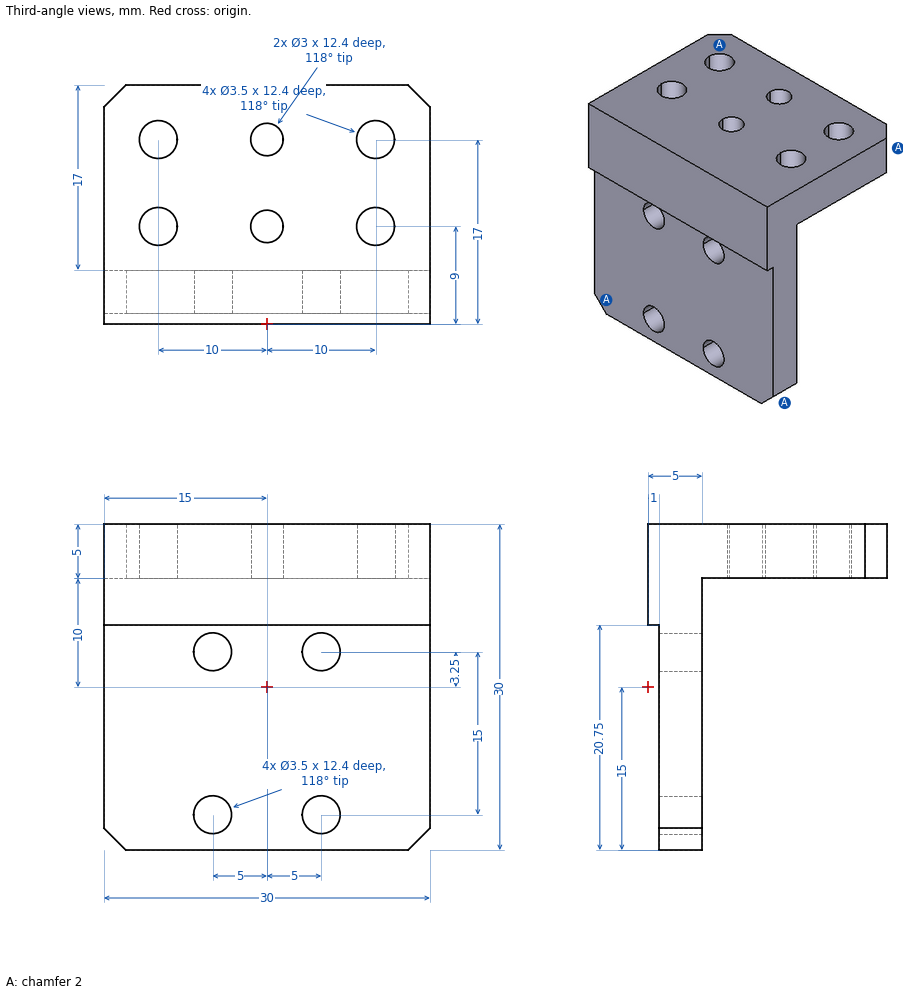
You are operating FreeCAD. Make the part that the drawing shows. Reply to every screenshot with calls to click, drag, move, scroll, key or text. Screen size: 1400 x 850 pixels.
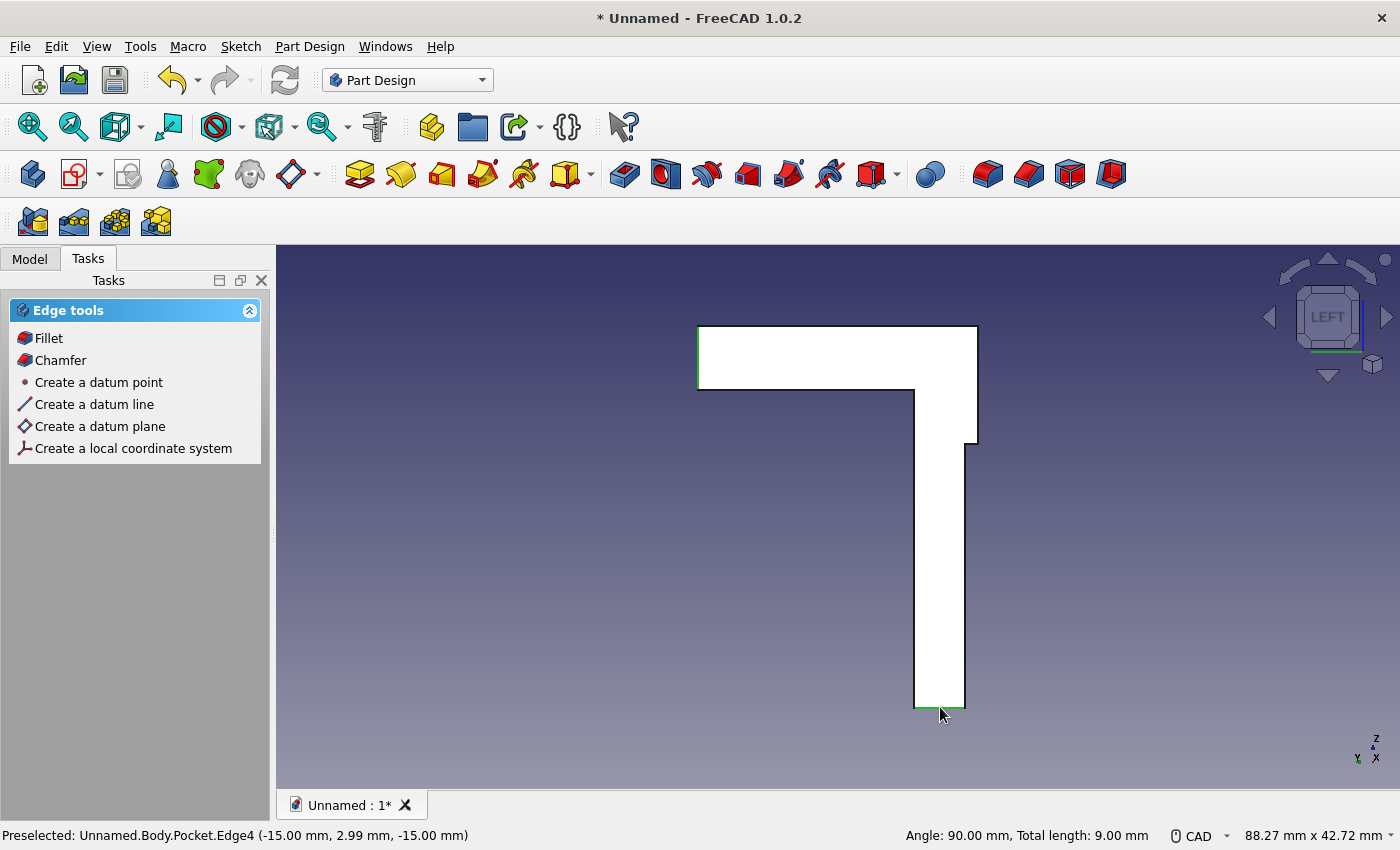
key(0)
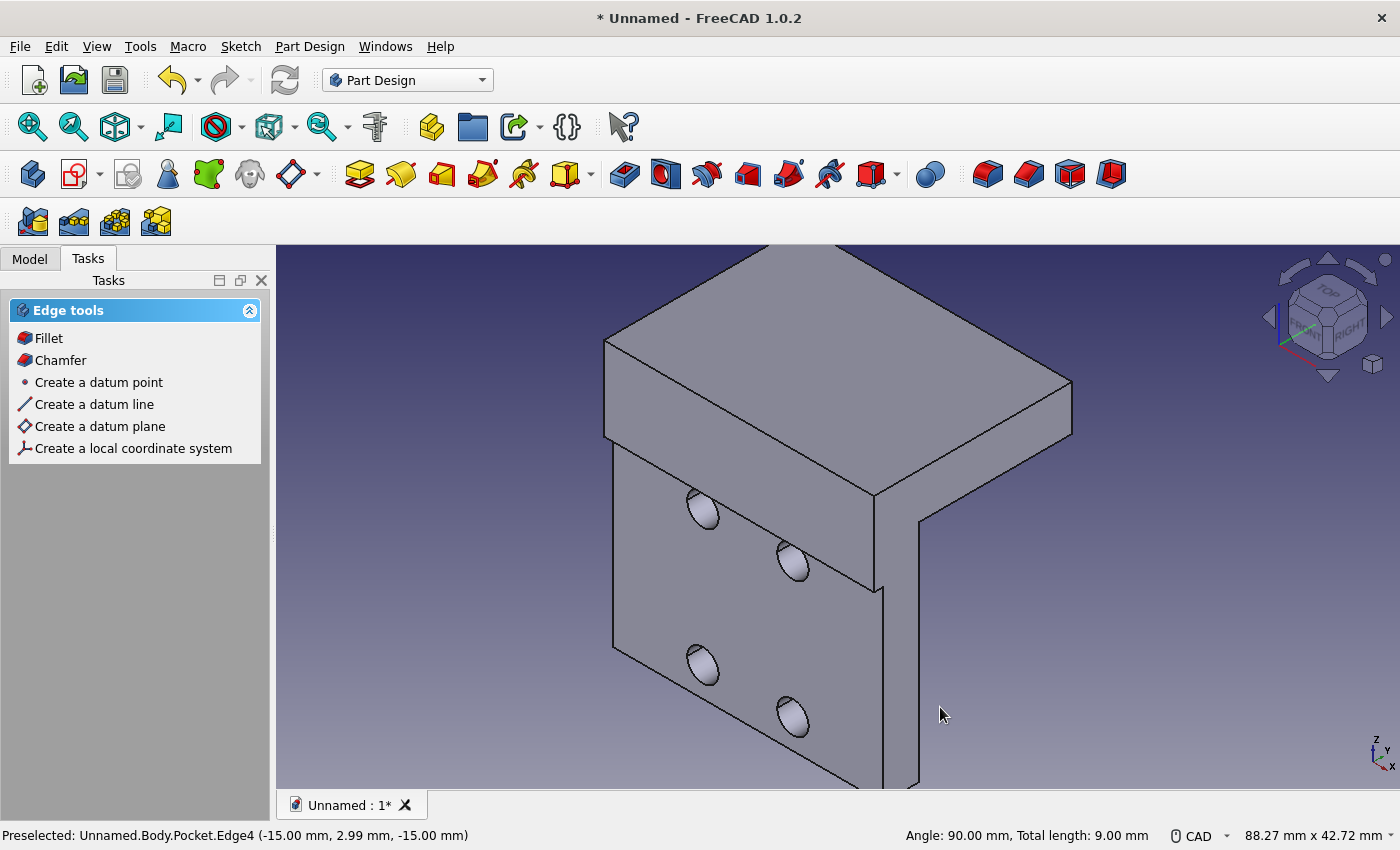
key(v)
key(f)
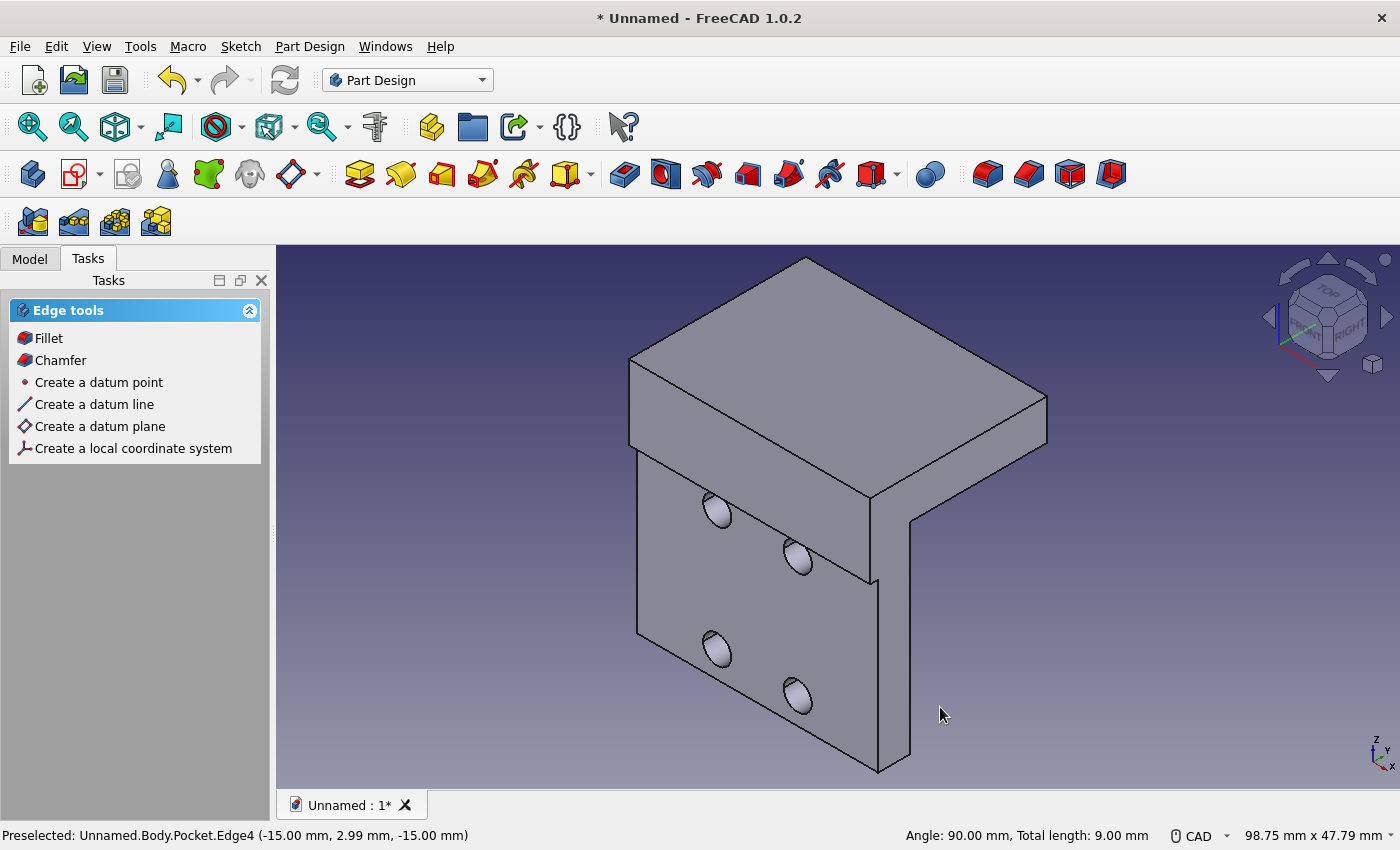
key(2)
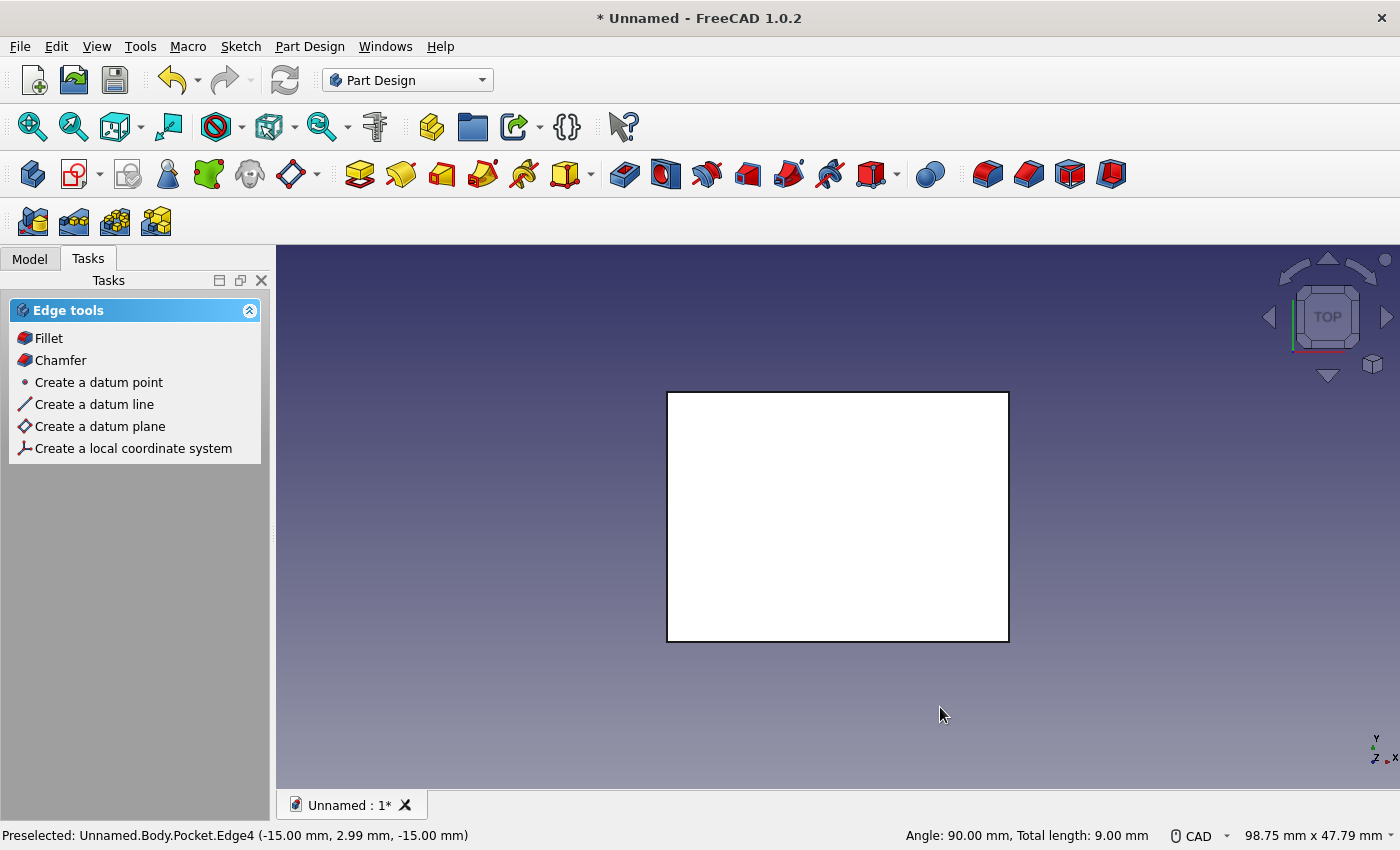
key(1)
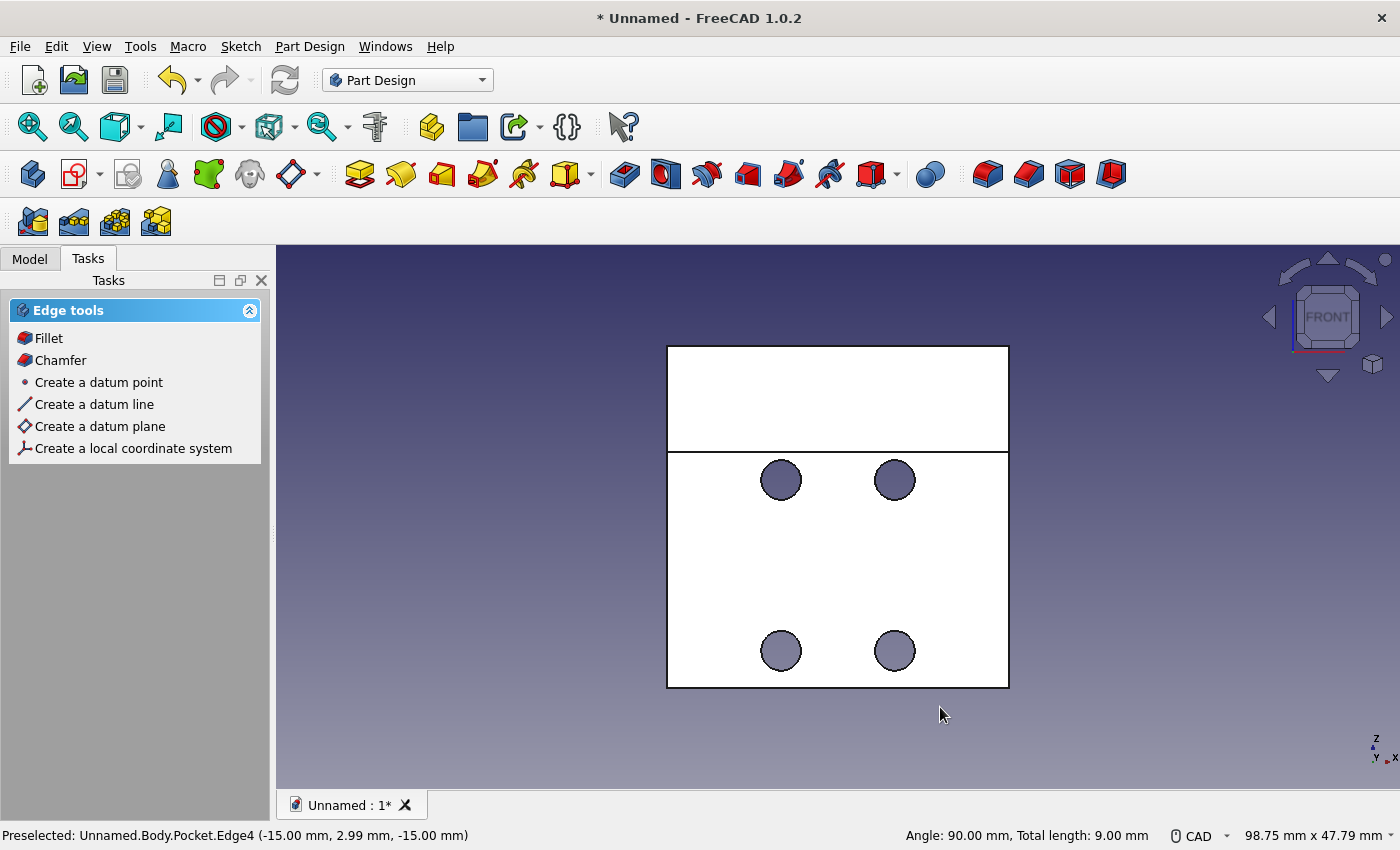
key(3)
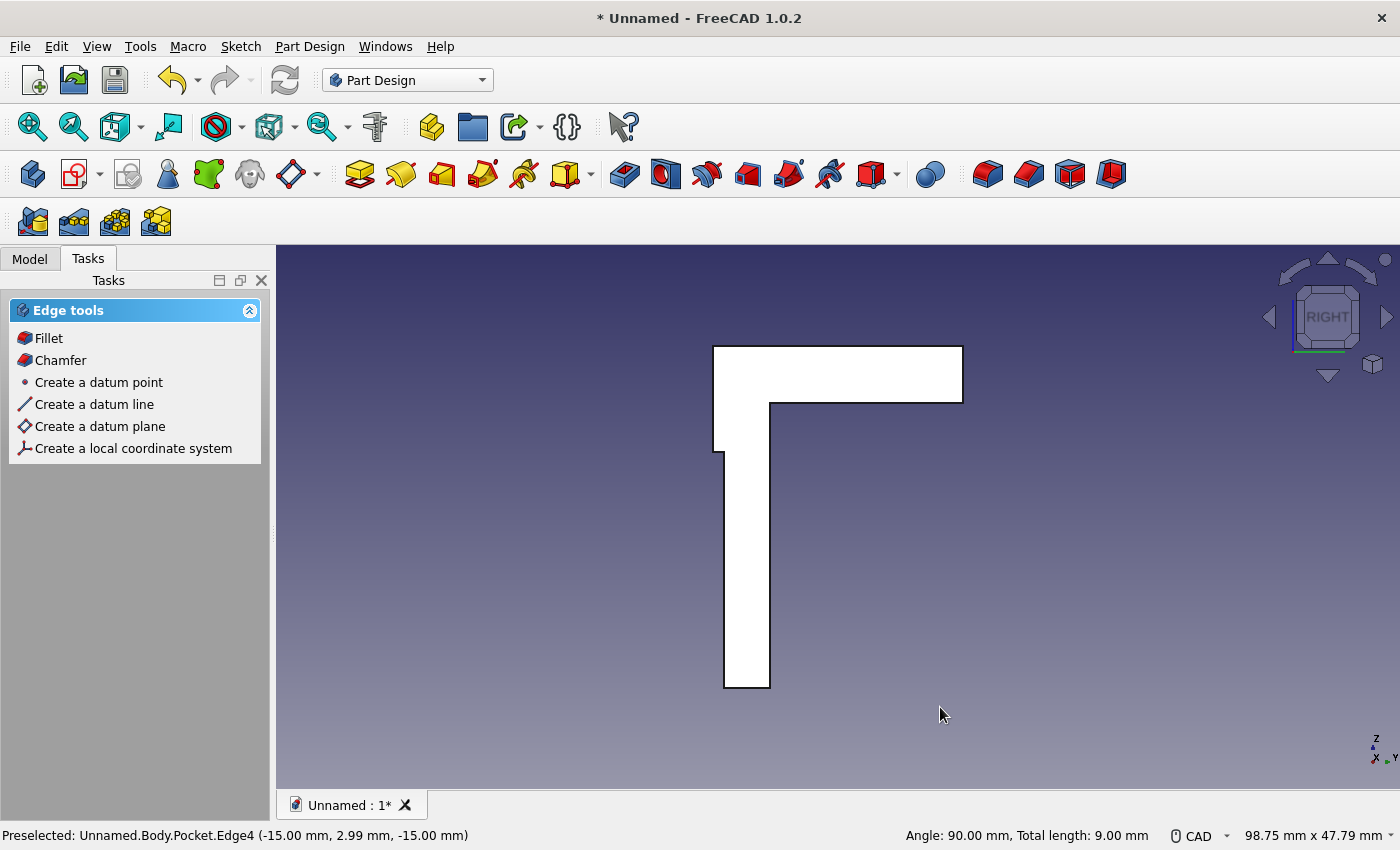
click(963, 374, ctrl)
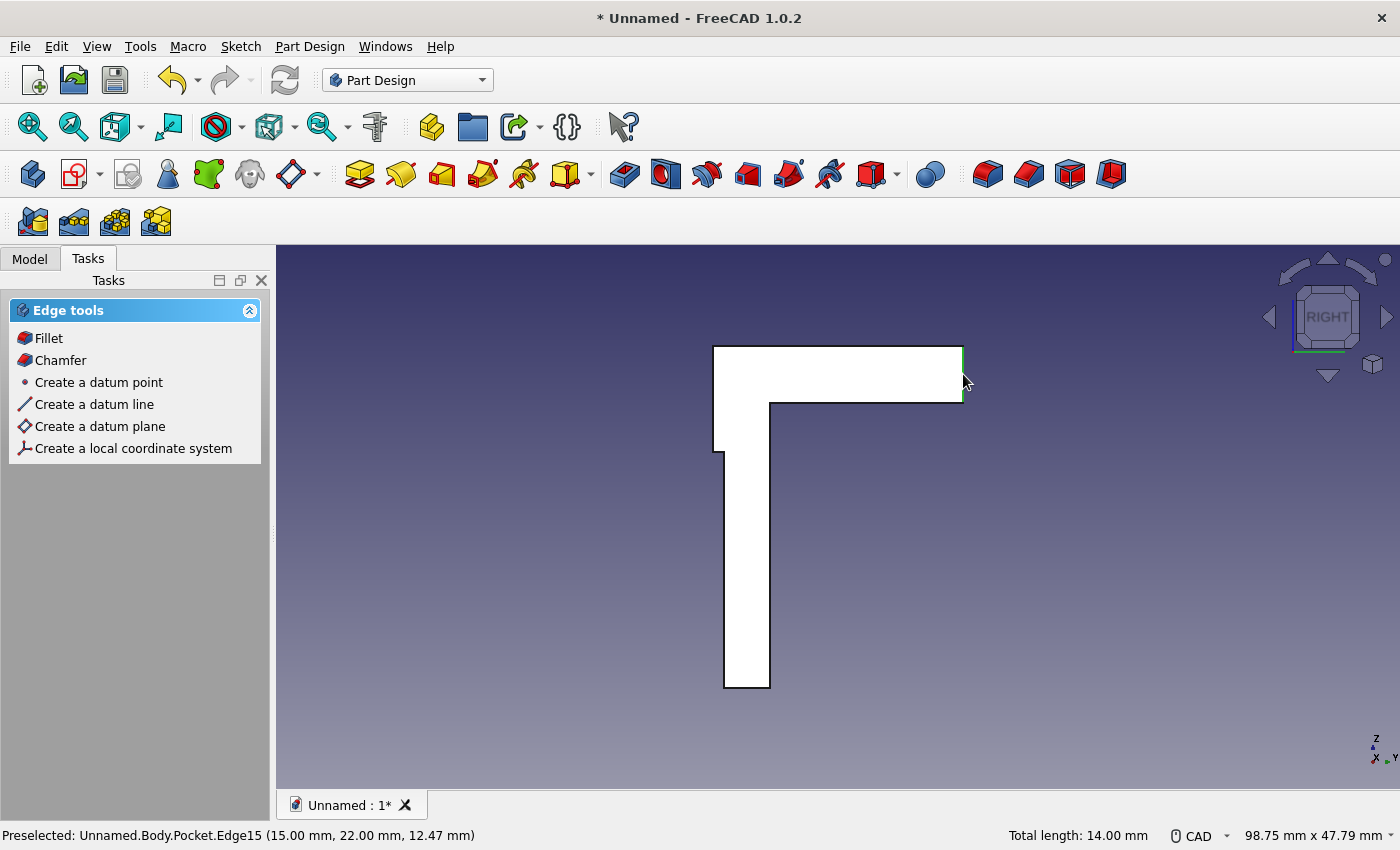
click(747, 687, ctrl)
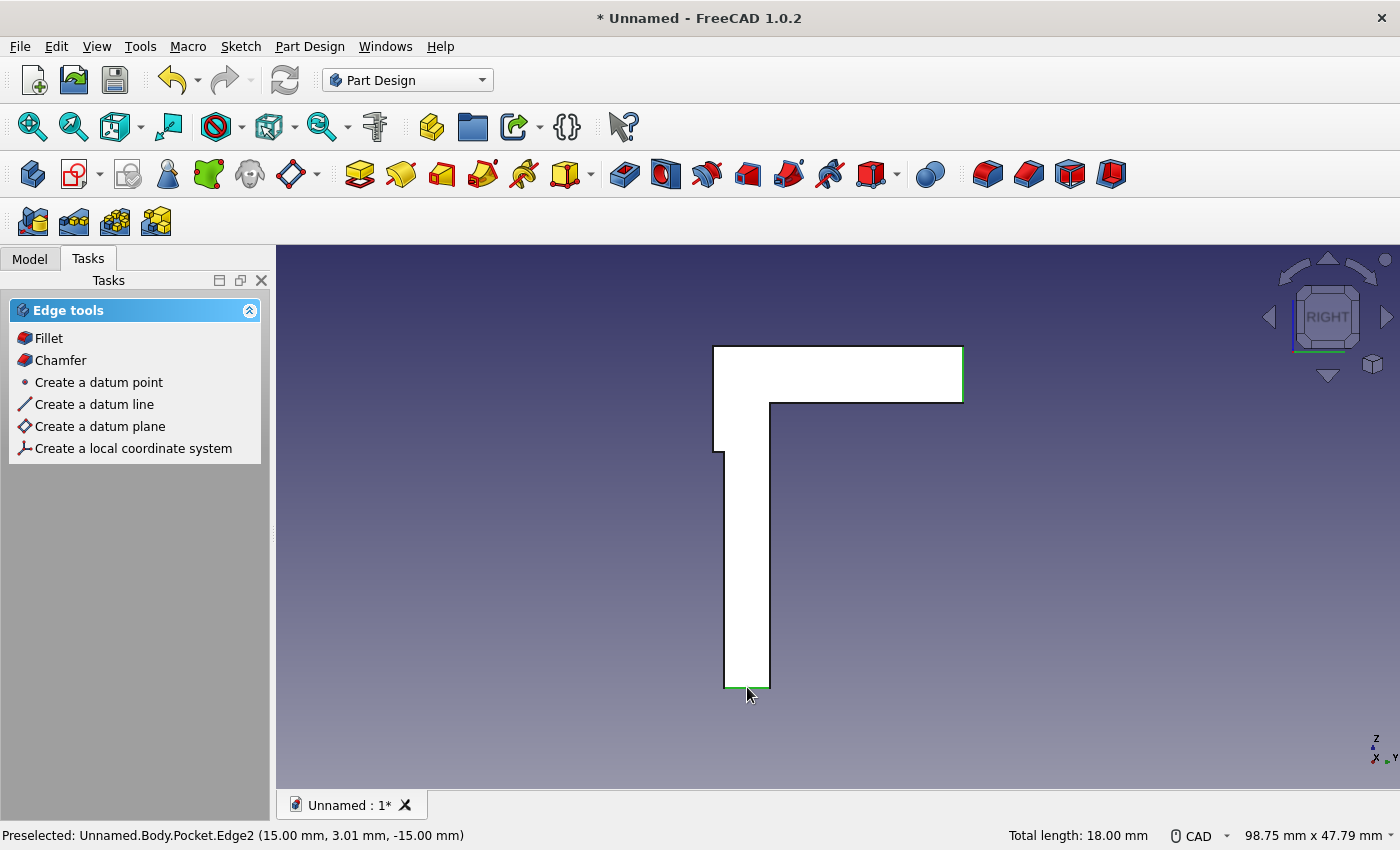
click(1029, 174)